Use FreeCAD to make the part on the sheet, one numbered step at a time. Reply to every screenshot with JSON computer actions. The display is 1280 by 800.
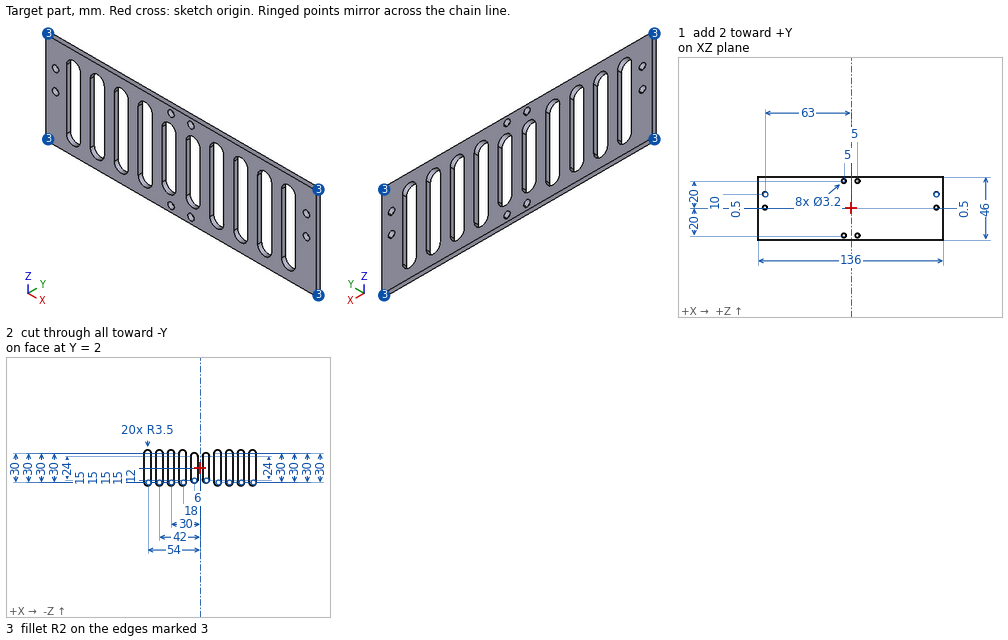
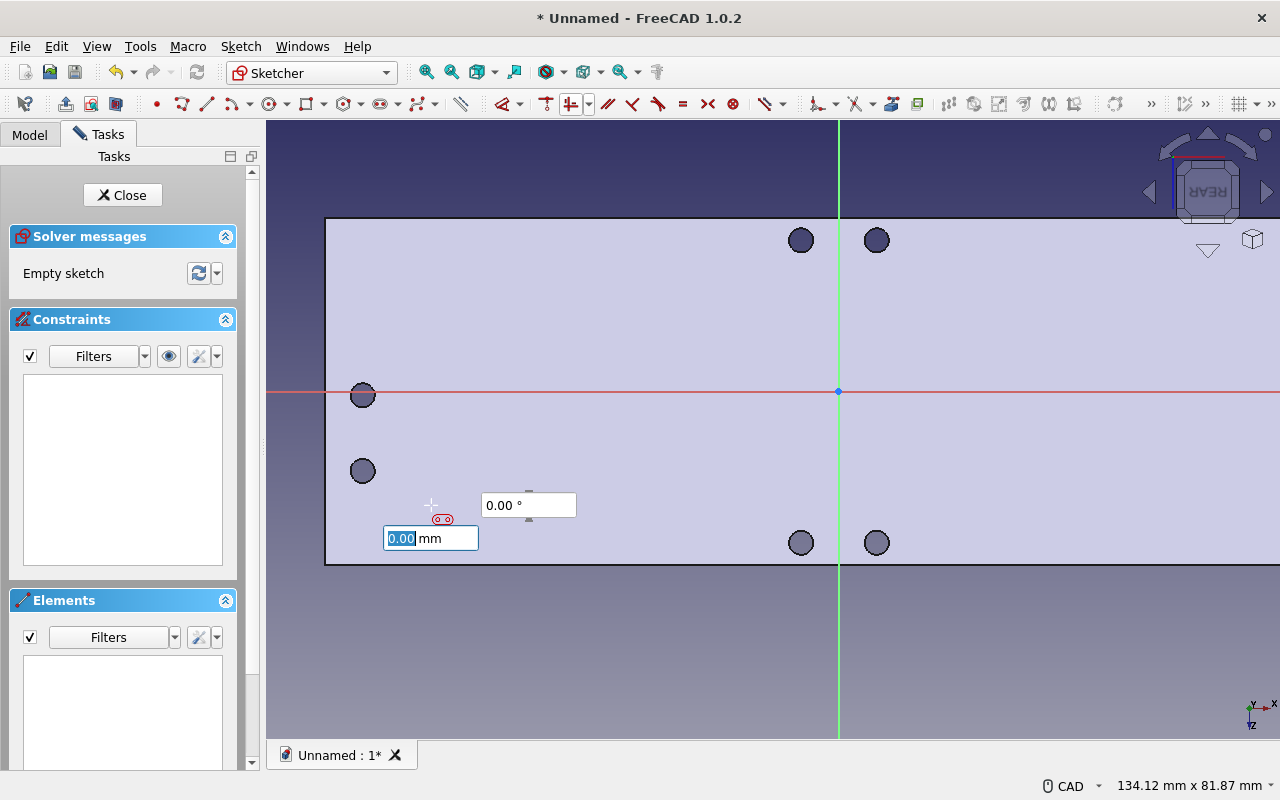
{"action": "left_click", "coordinate": [431, 278]}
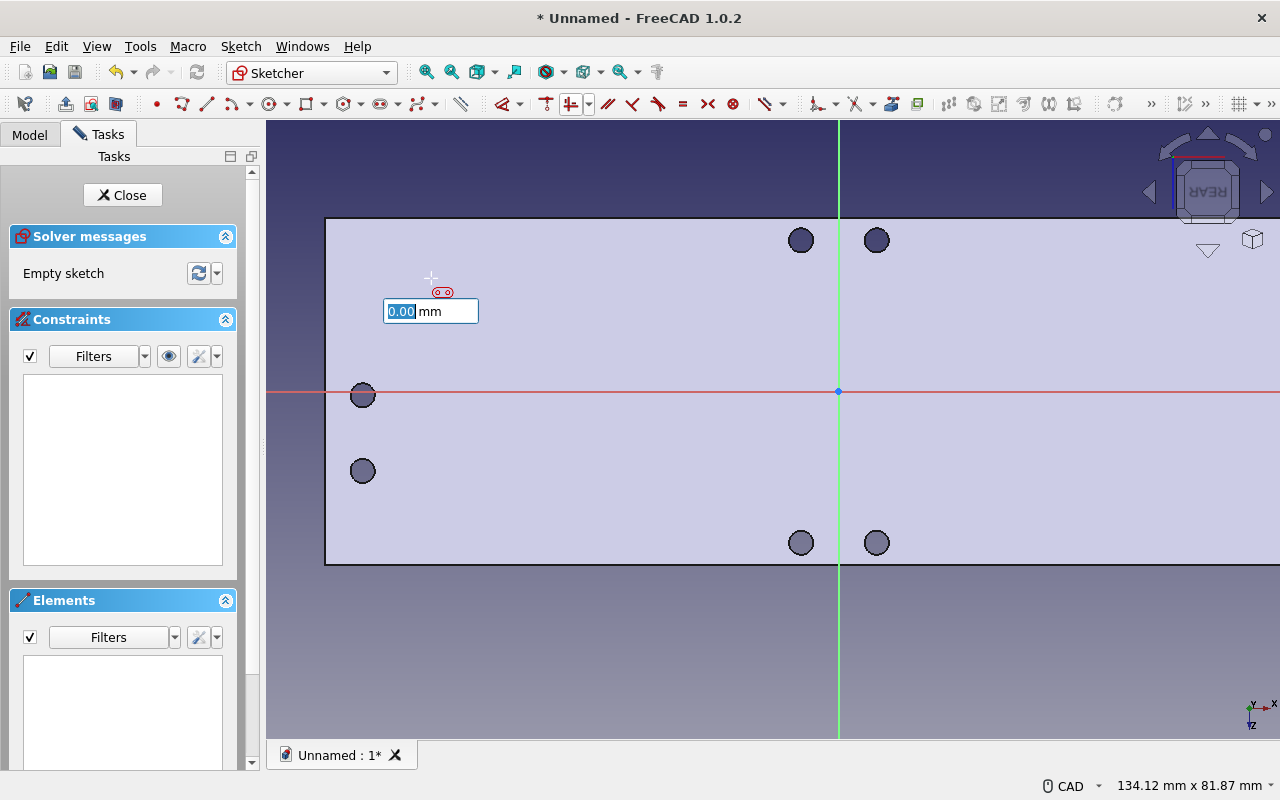
{"action": "left_click", "coordinate": [457, 426]}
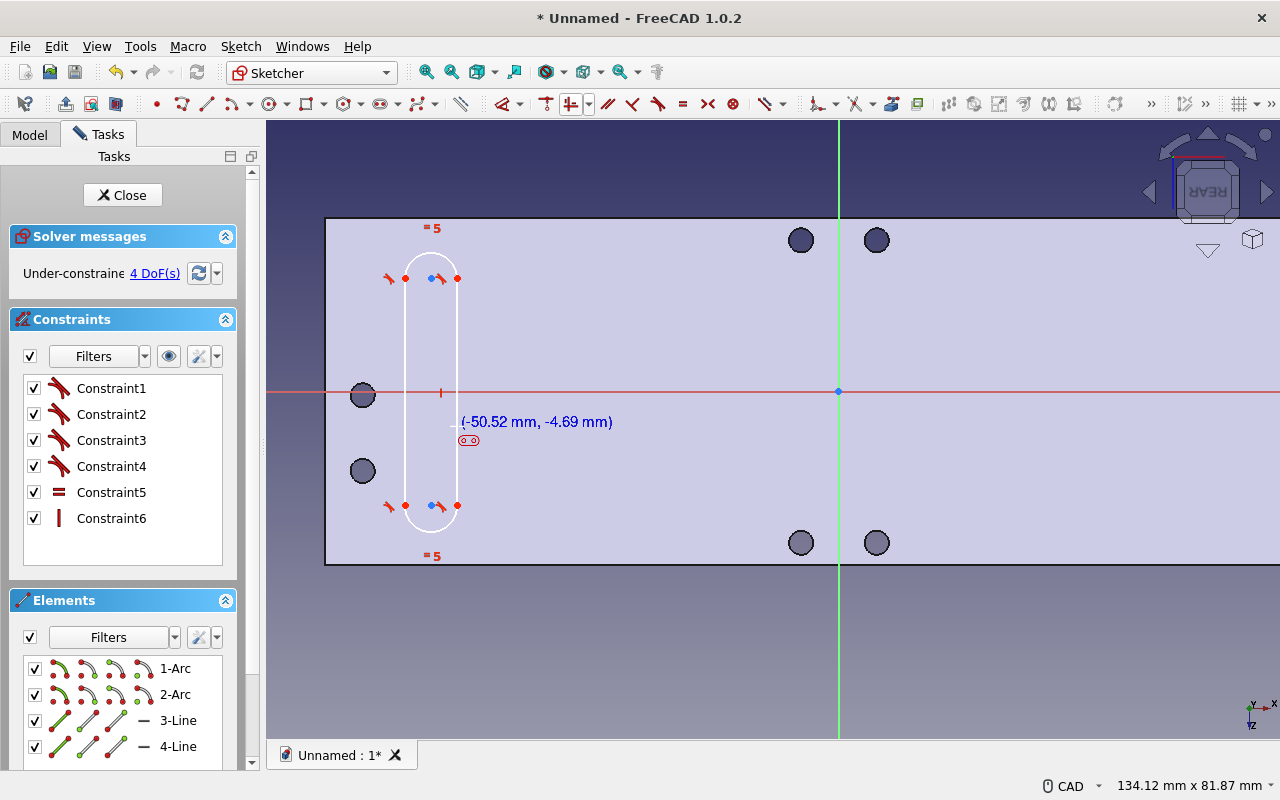
{"action": "left_click", "coordinate": [521, 505]}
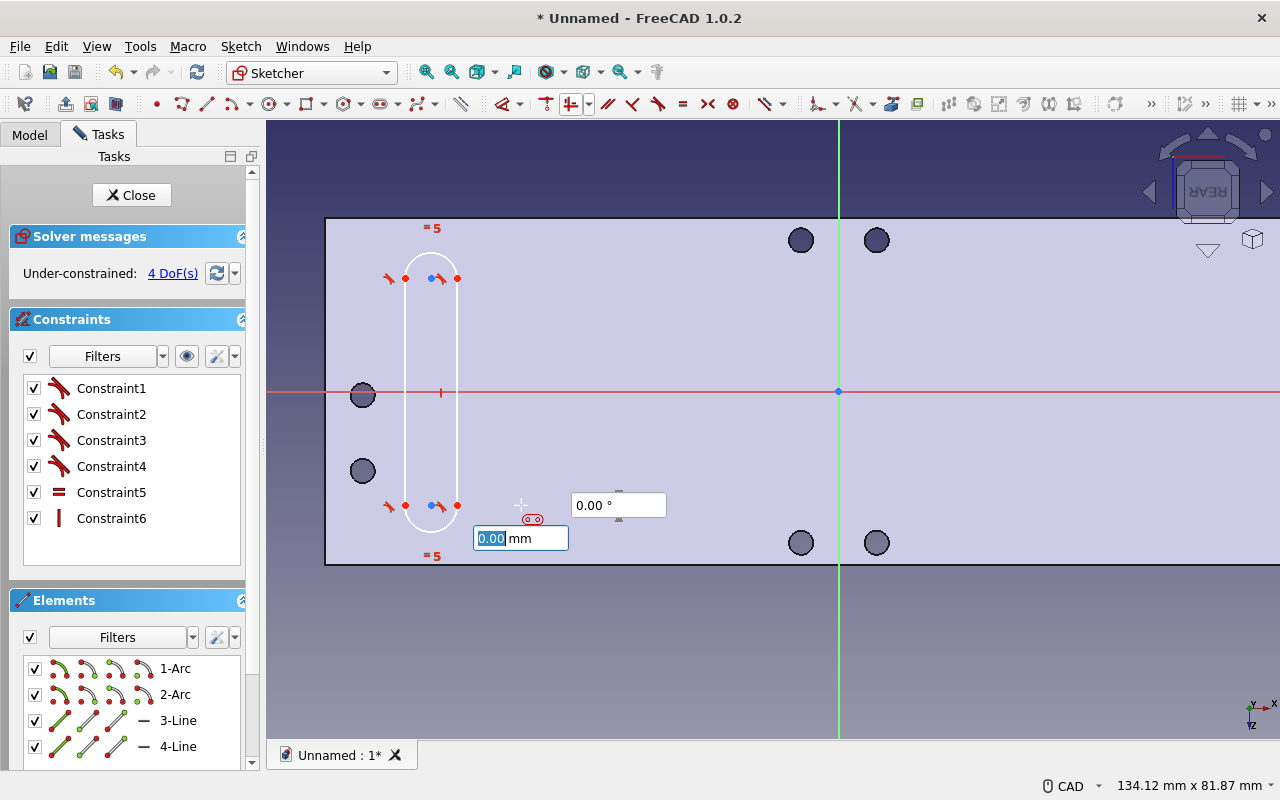
{"action": "left_click", "coordinate": [521, 278]}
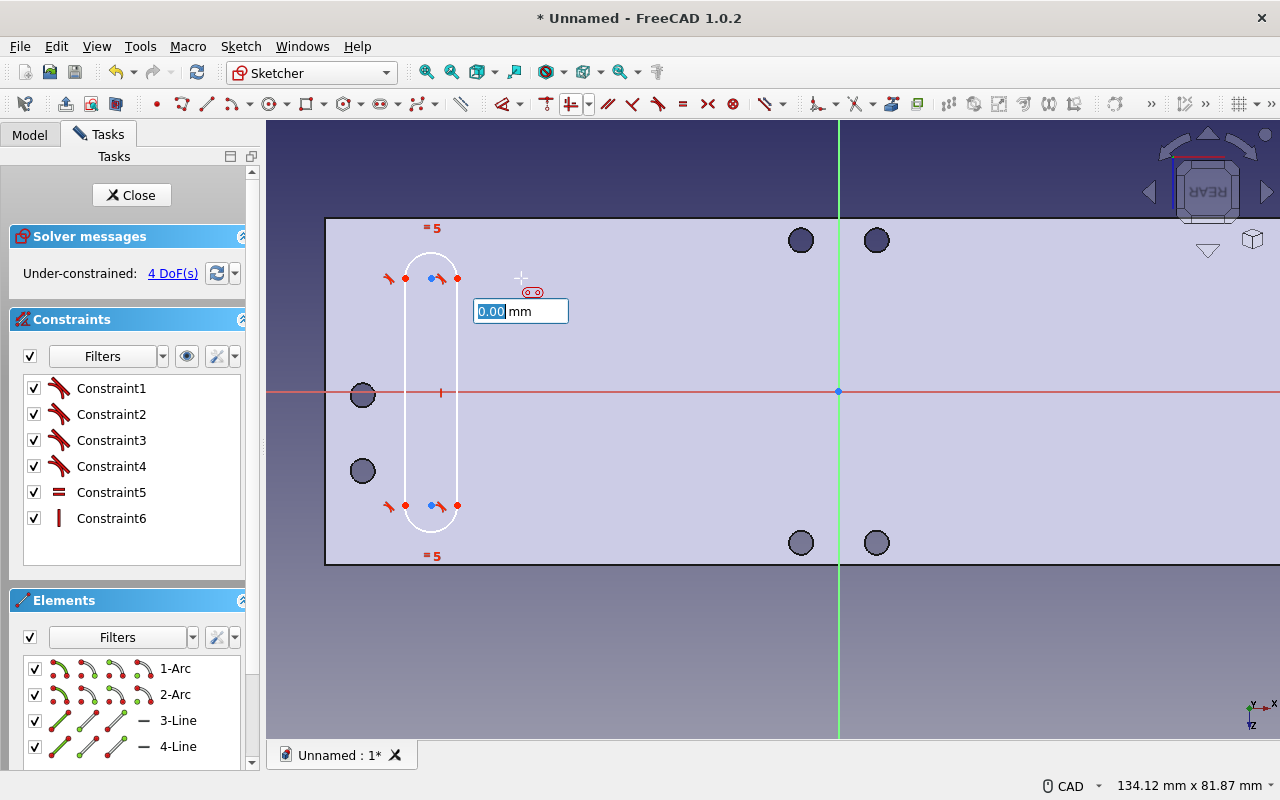
{"action": "left_click", "coordinate": [548, 426]}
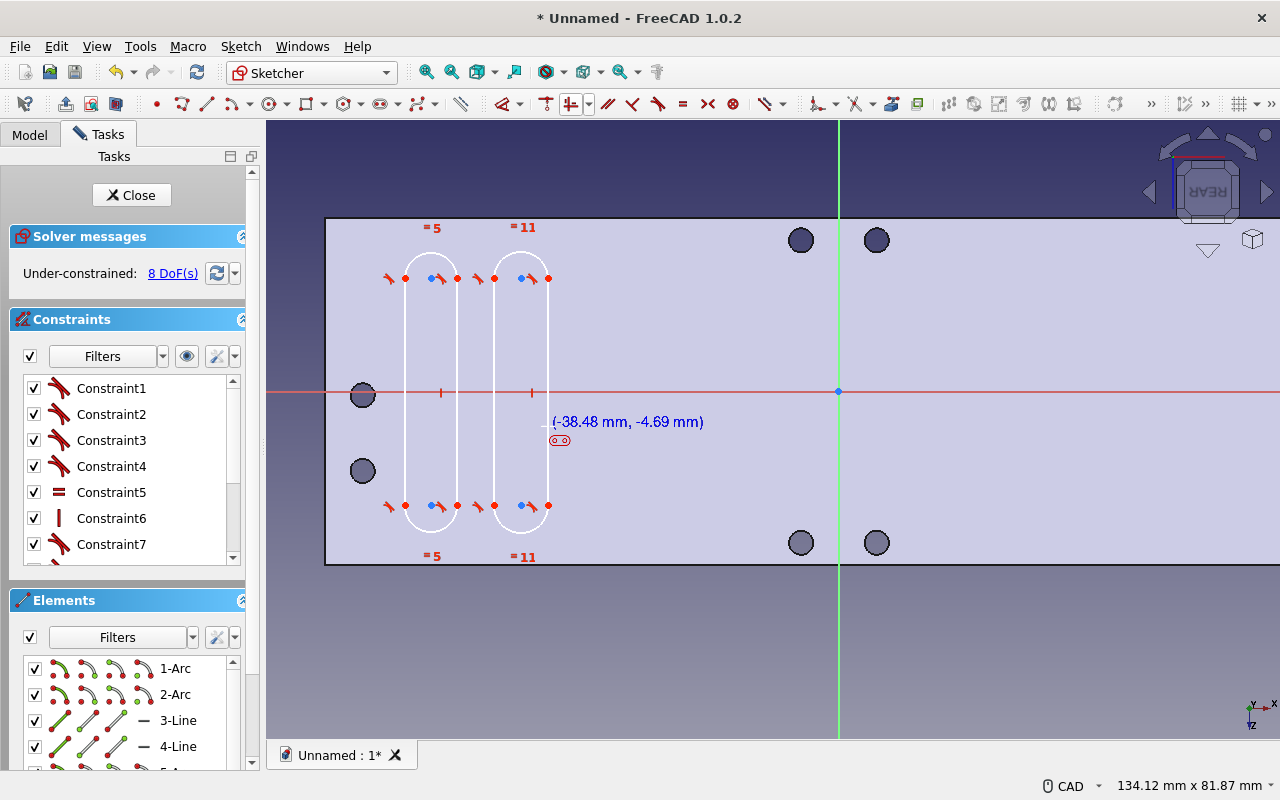
{"action": "left_click", "coordinate": [612, 505]}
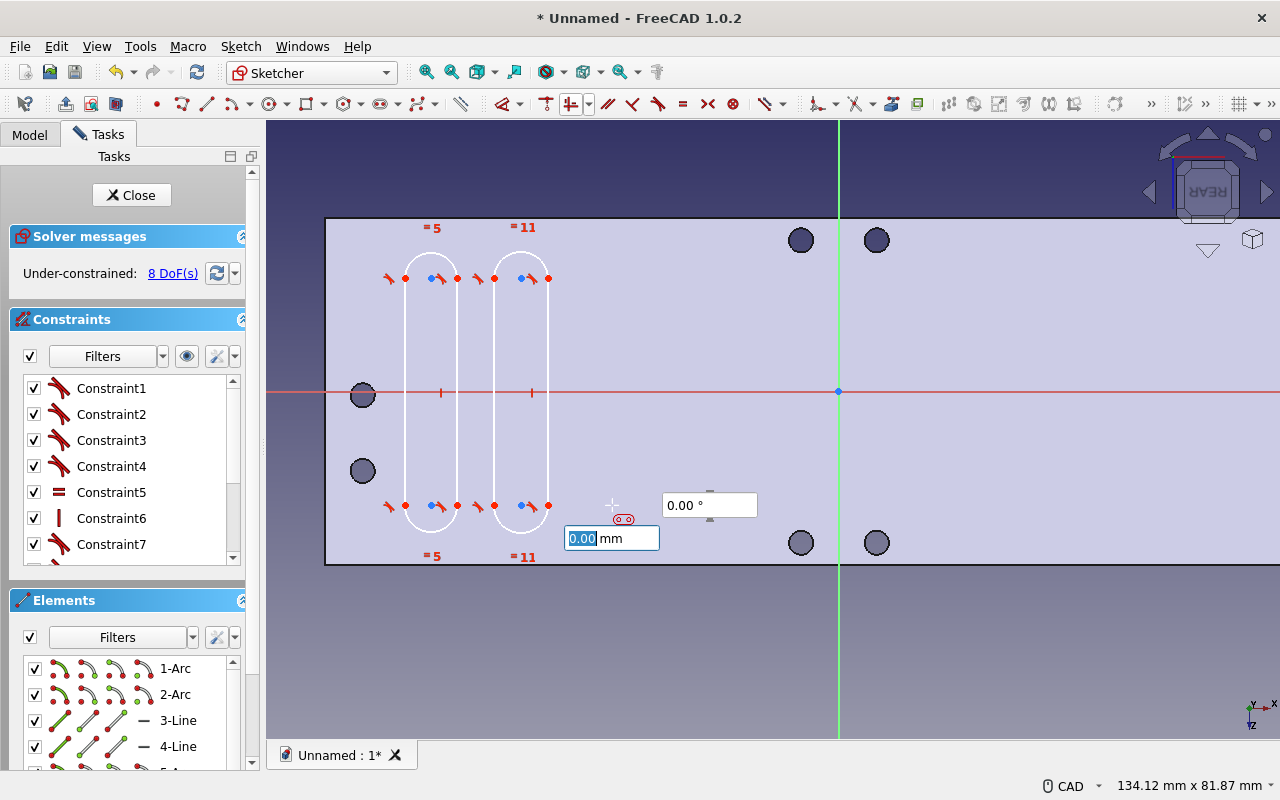
{"action": "left_click", "coordinate": [612, 278]}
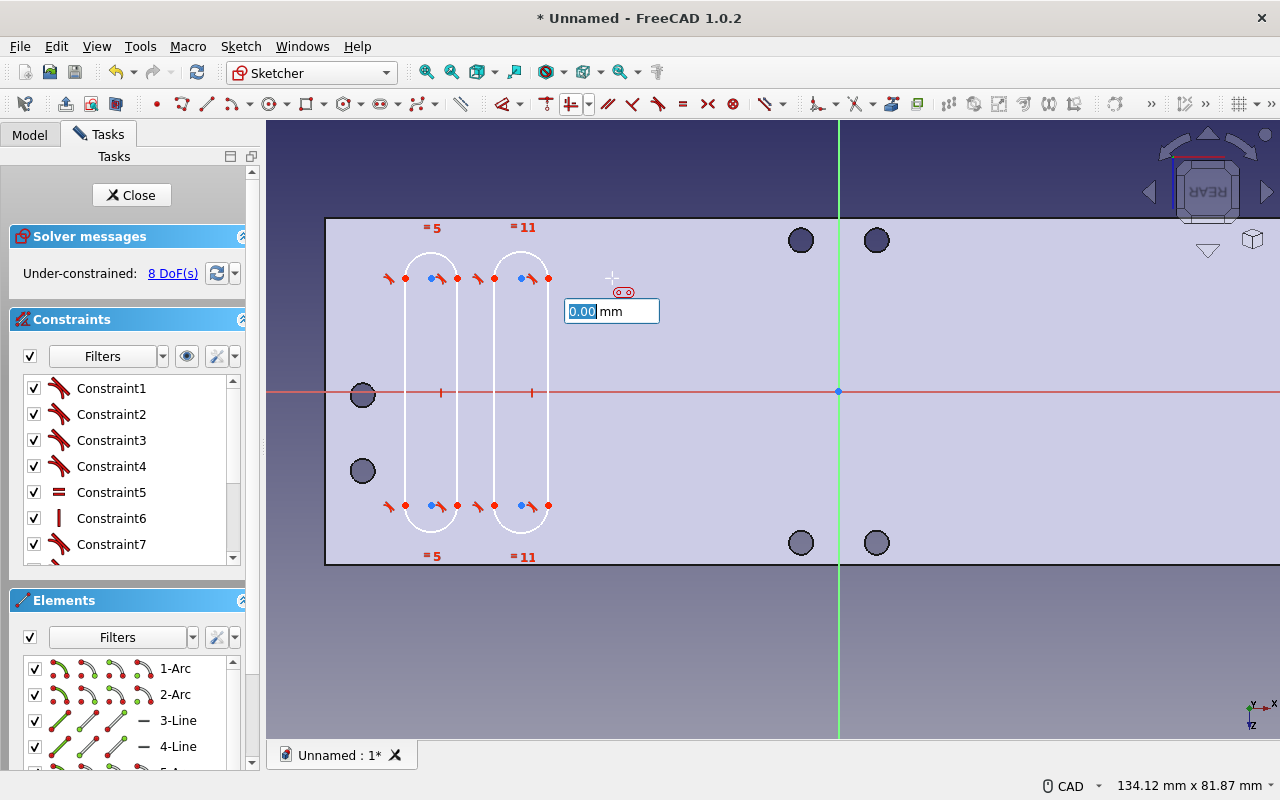
{"action": "left_click", "coordinate": [639, 426]}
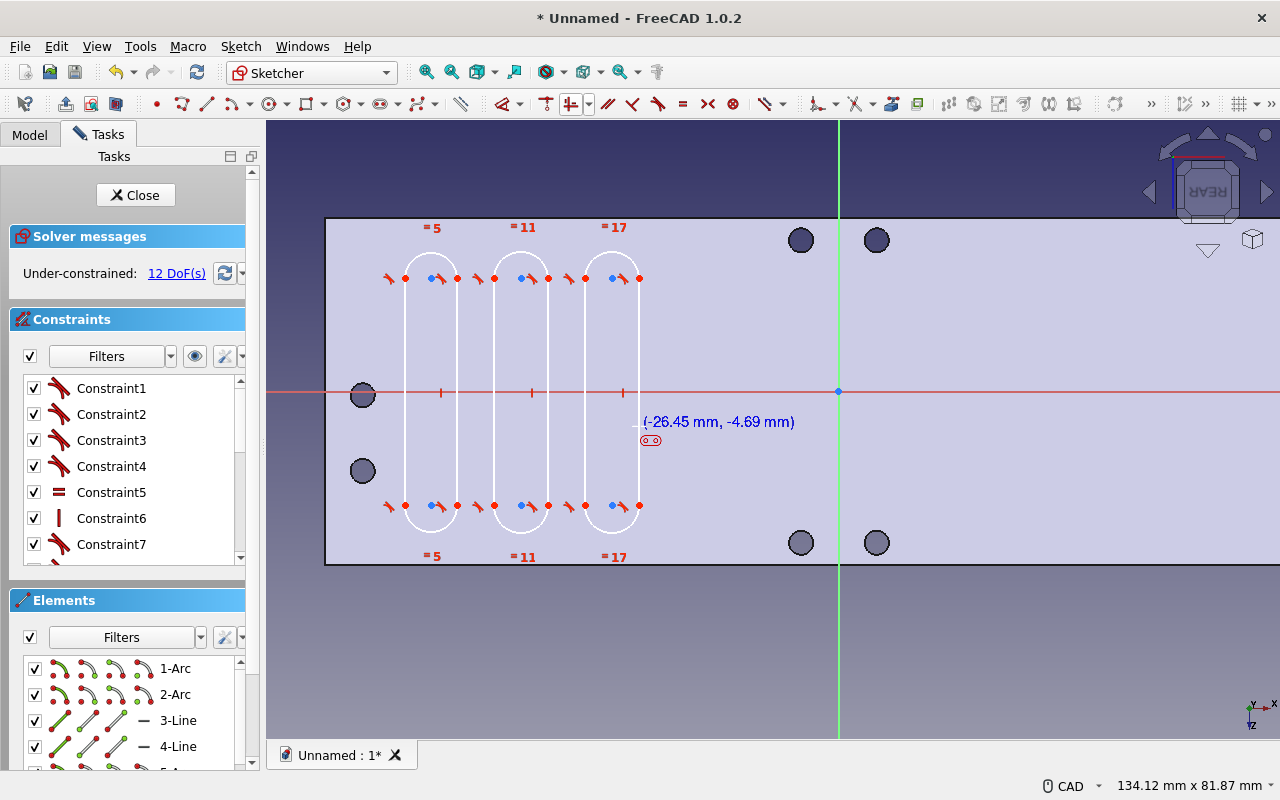
{"action": "left_click", "coordinate": [703, 505]}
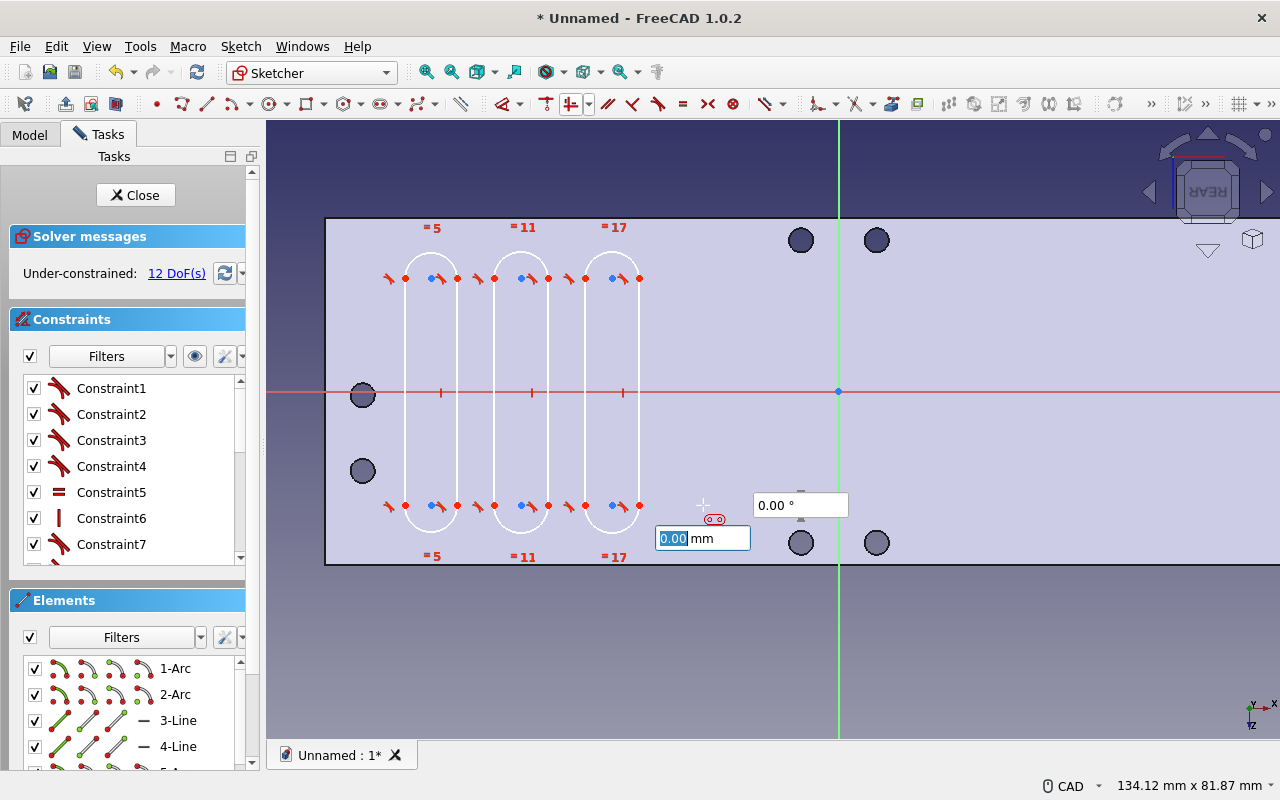
{"action": "left_click", "coordinate": [703, 278]}